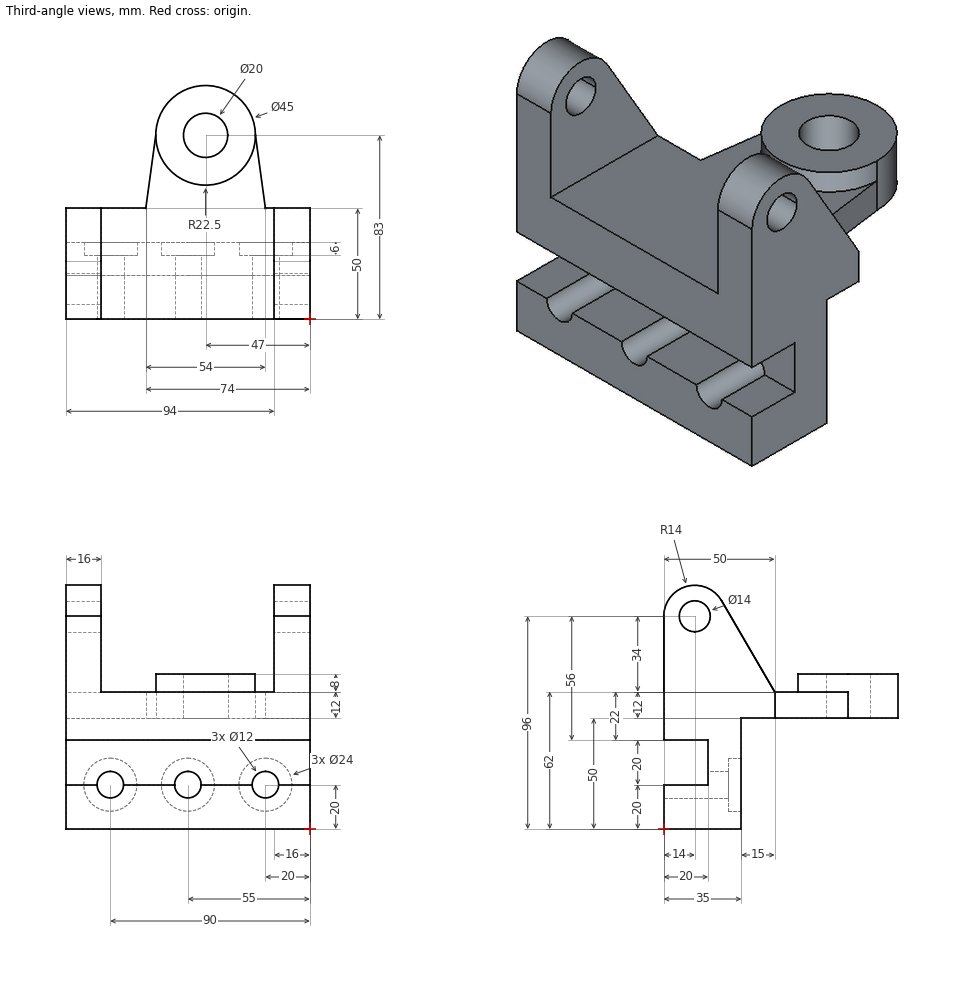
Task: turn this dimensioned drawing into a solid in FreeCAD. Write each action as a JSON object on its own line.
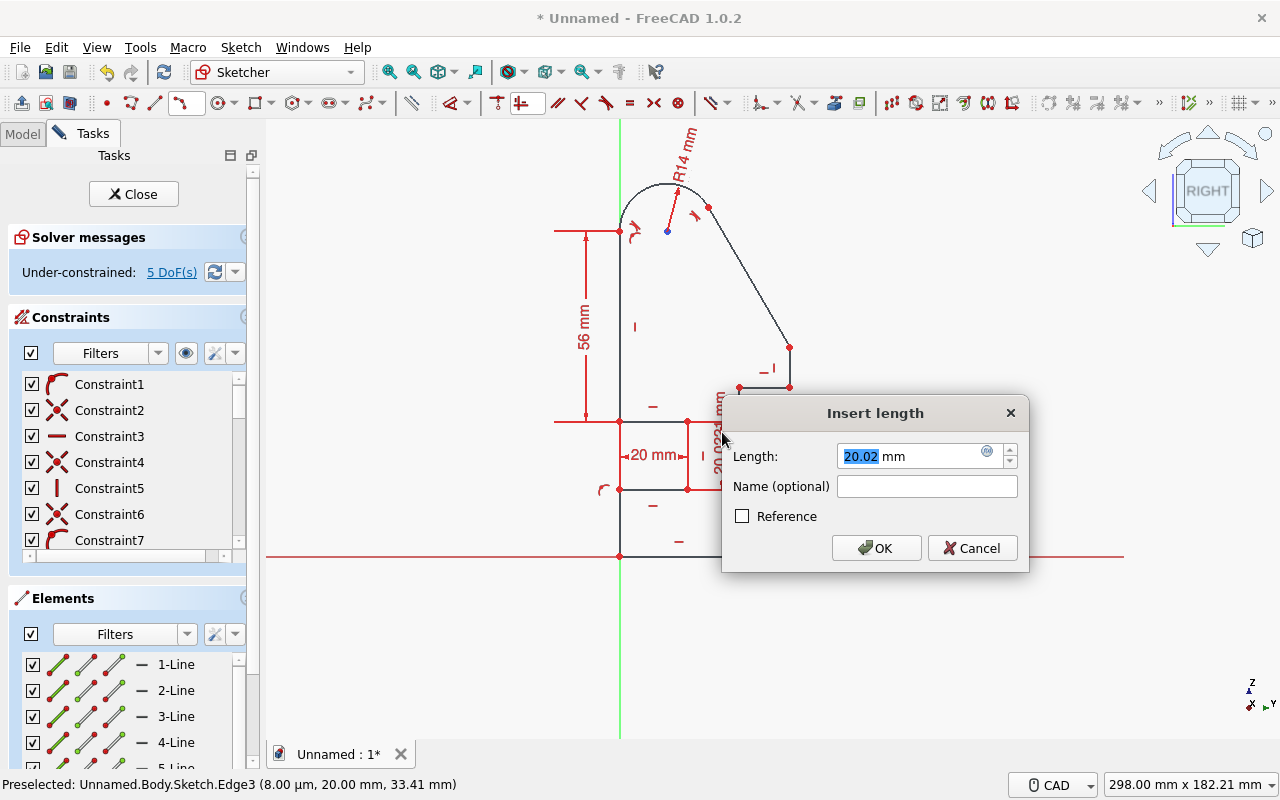
{"action": "type", "text": "20"}
{"action": "key", "text": "Return"}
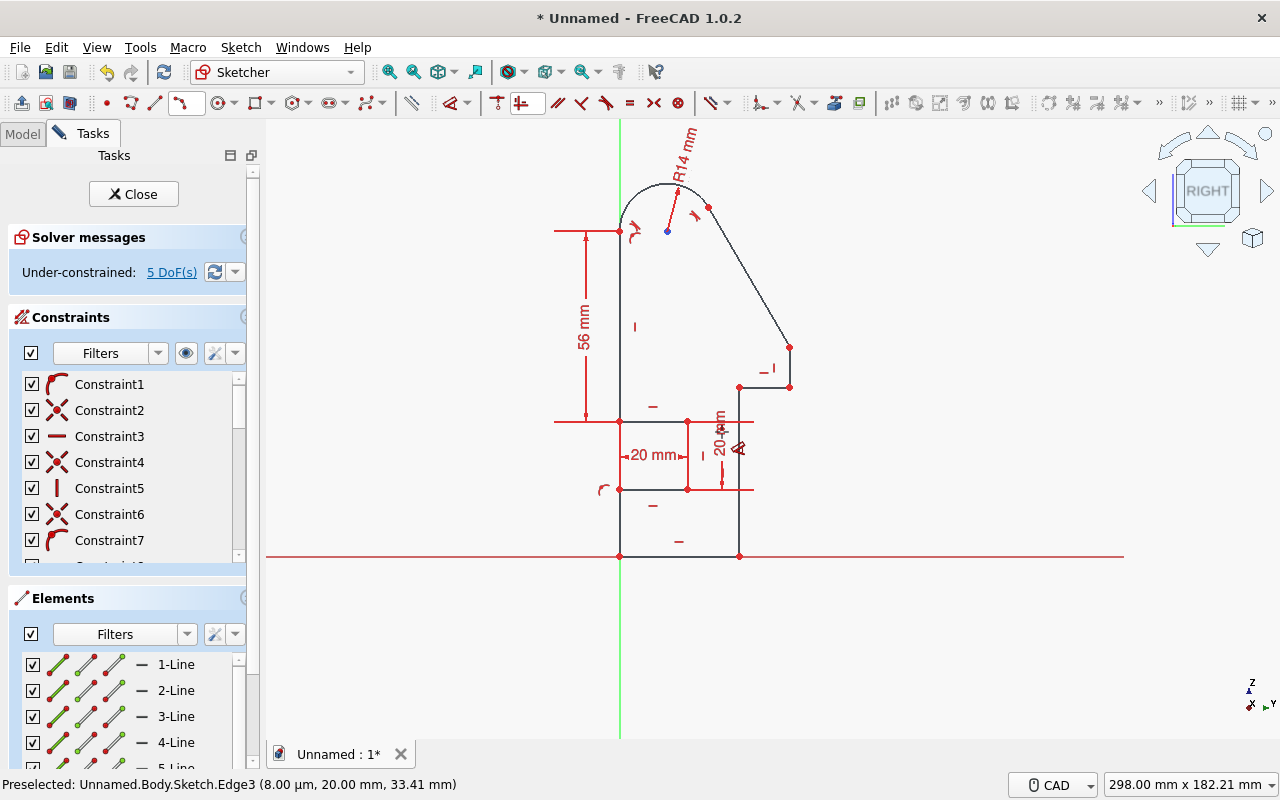
{"action": "left_click", "coordinate": [620, 510]}
{"action": "left_click", "coordinate": [586, 523]}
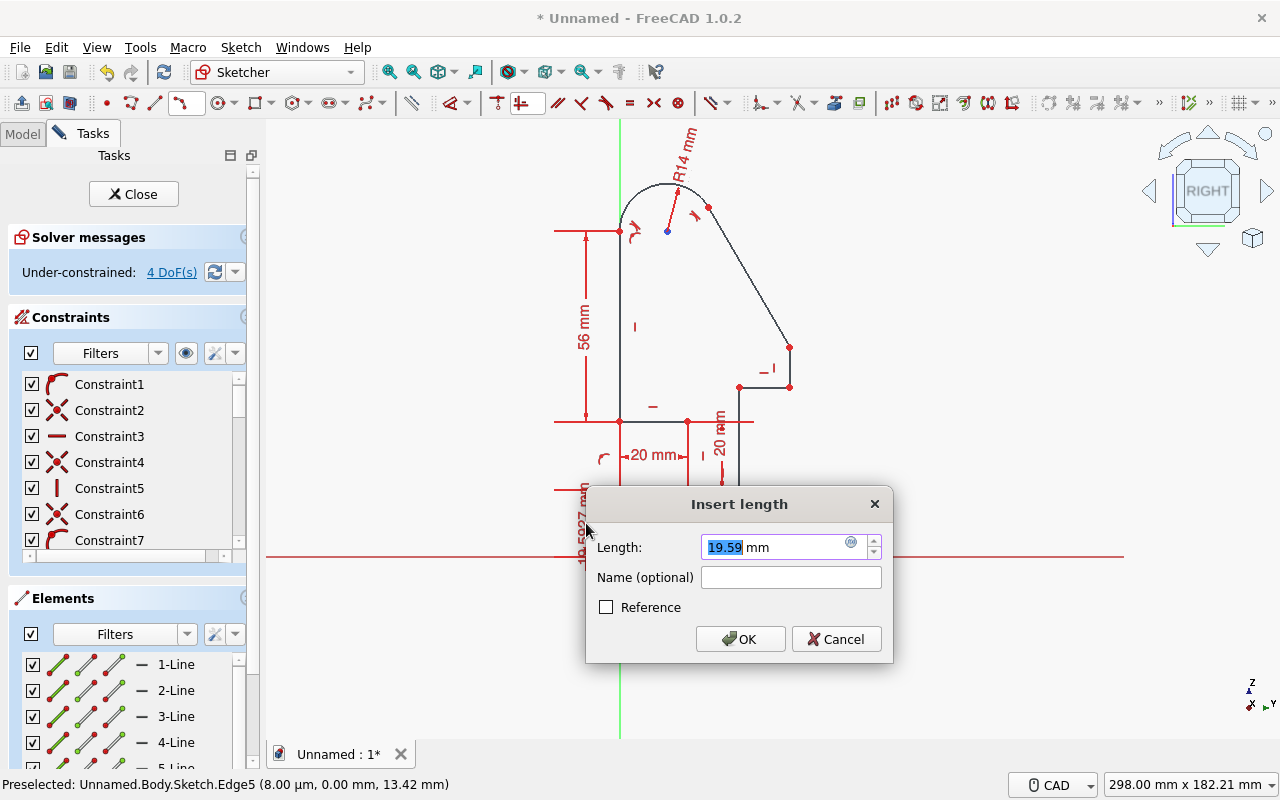
{"action": "type", "text": "20"}
{"action": "key", "text": "Return"}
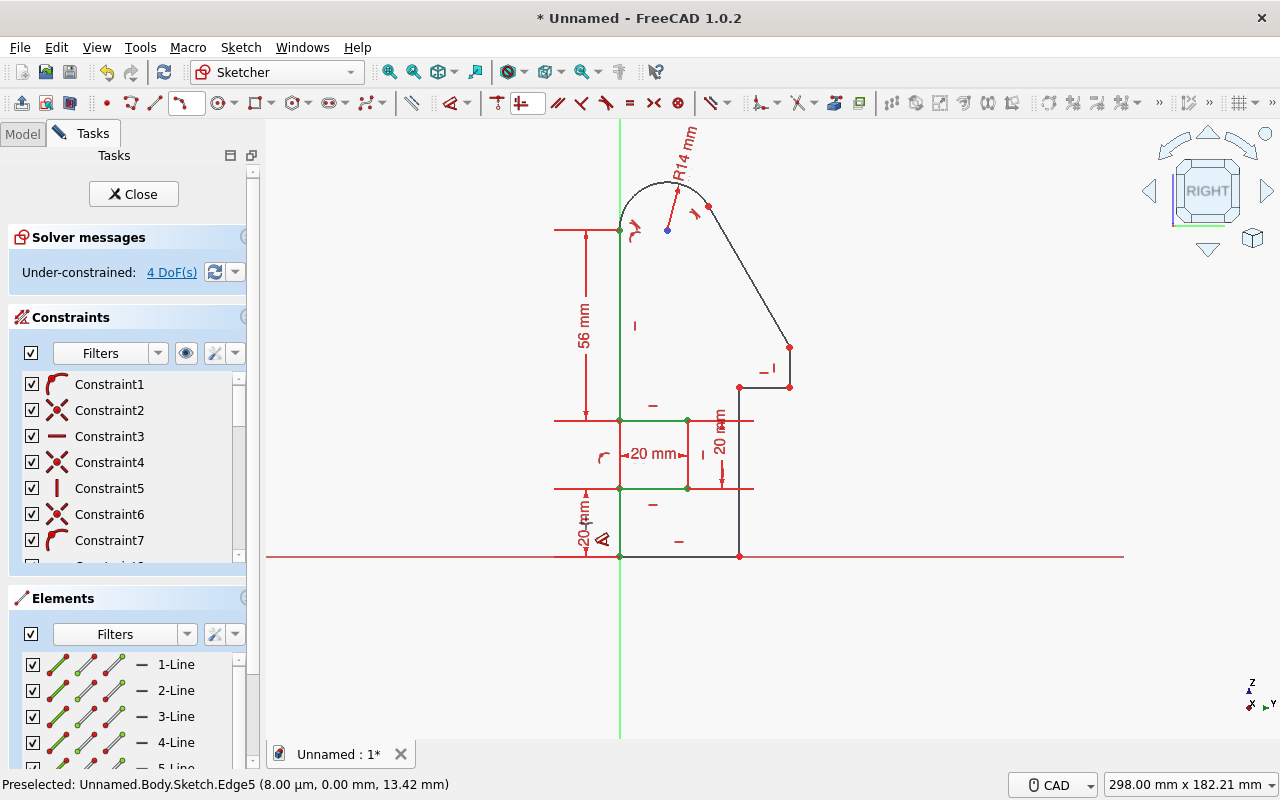
{"action": "left_click", "coordinate": [655, 557]}
{"action": "left_click", "coordinate": [679, 591]}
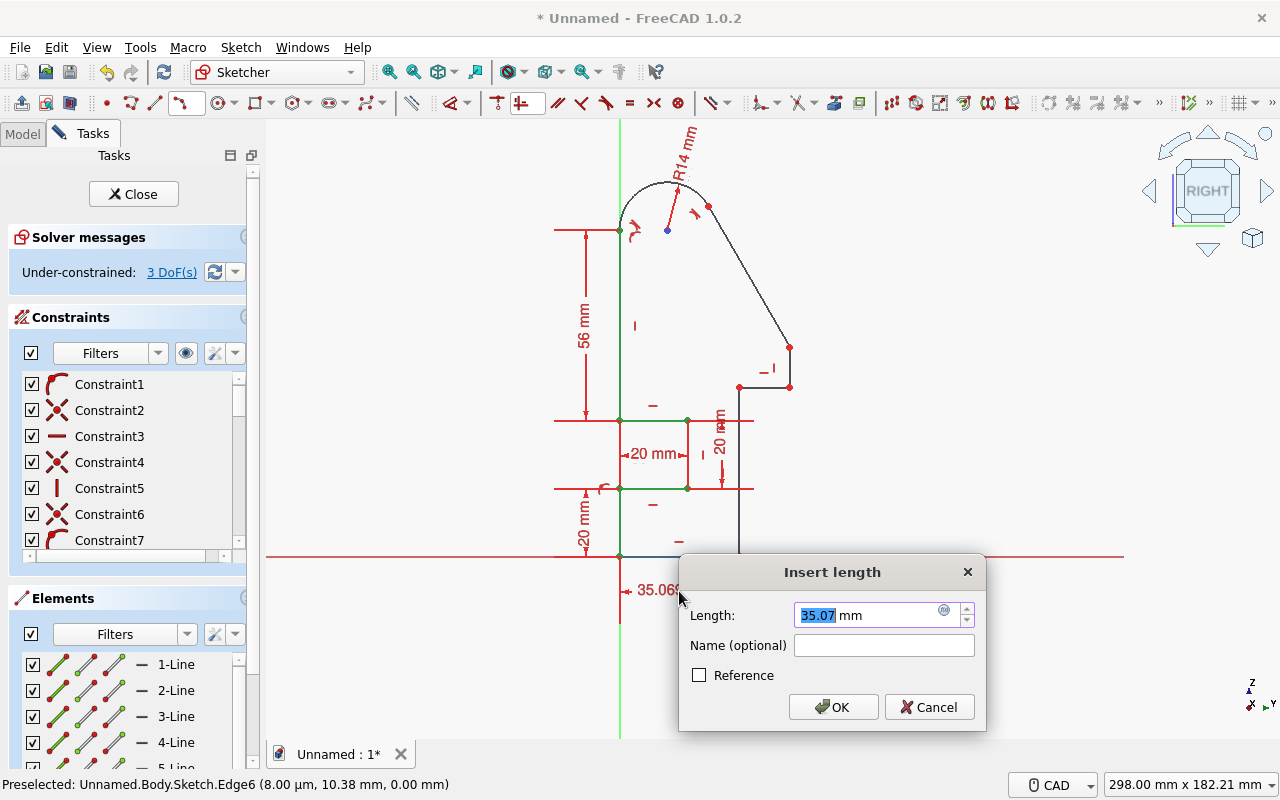
{"action": "type", "text": "35"}
{"action": "key", "text": "Return"}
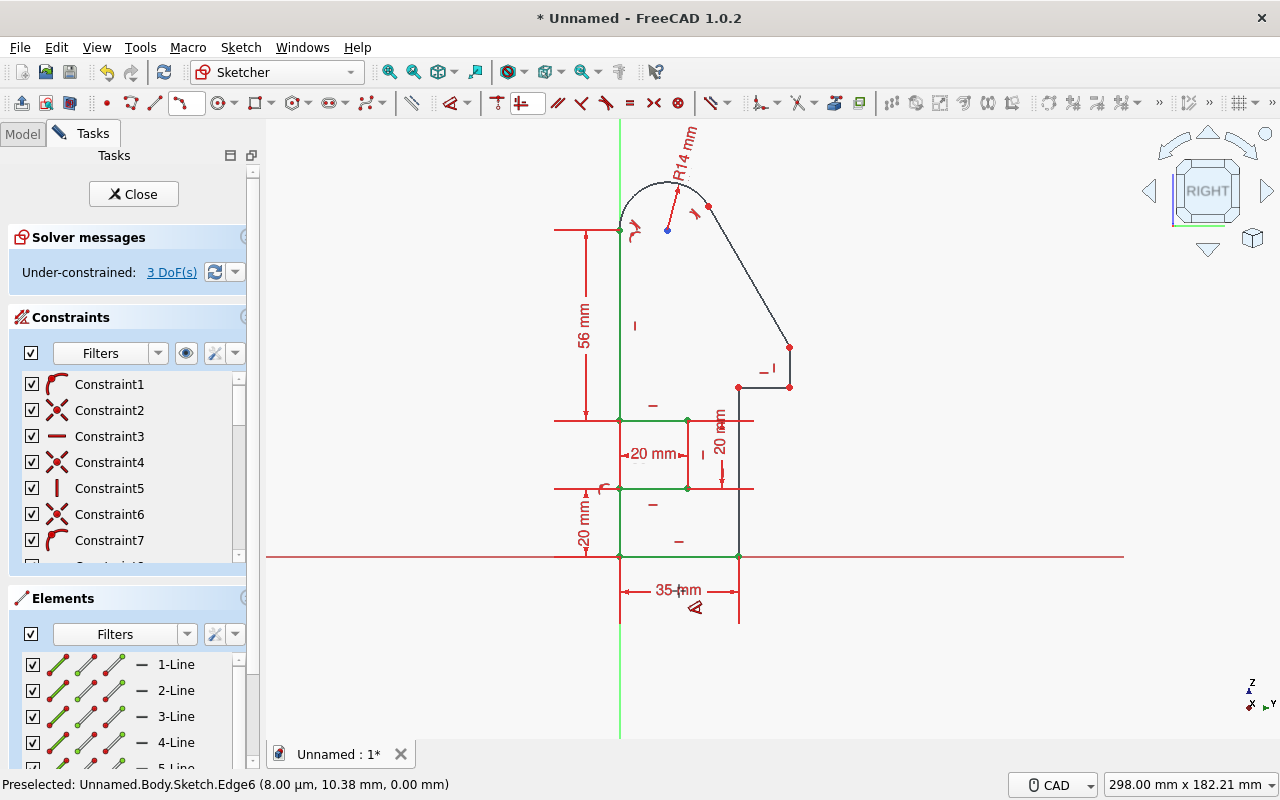
{"action": "left_click", "coordinate": [739, 506]}
{"action": "left_click", "coordinate": [773, 472]}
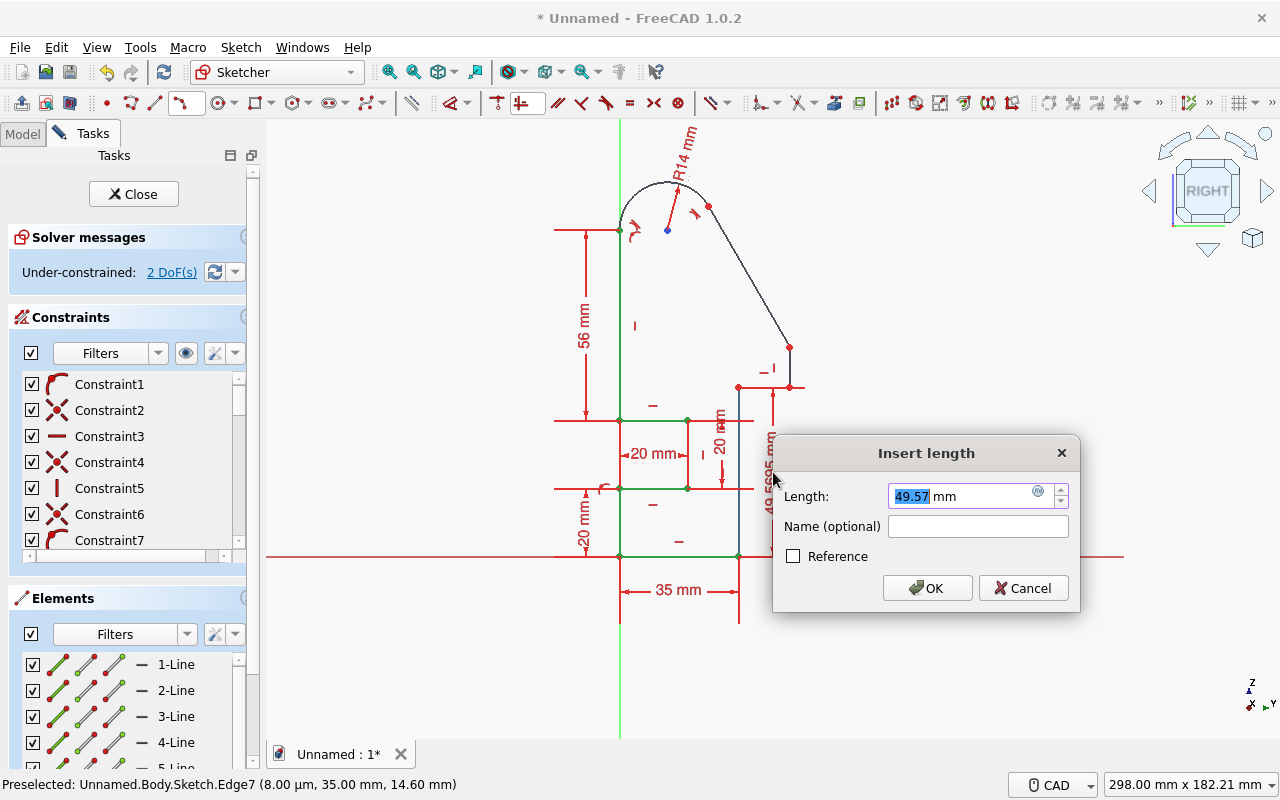
{"action": "type", "text": "50"}
{"action": "key", "text": "Return"}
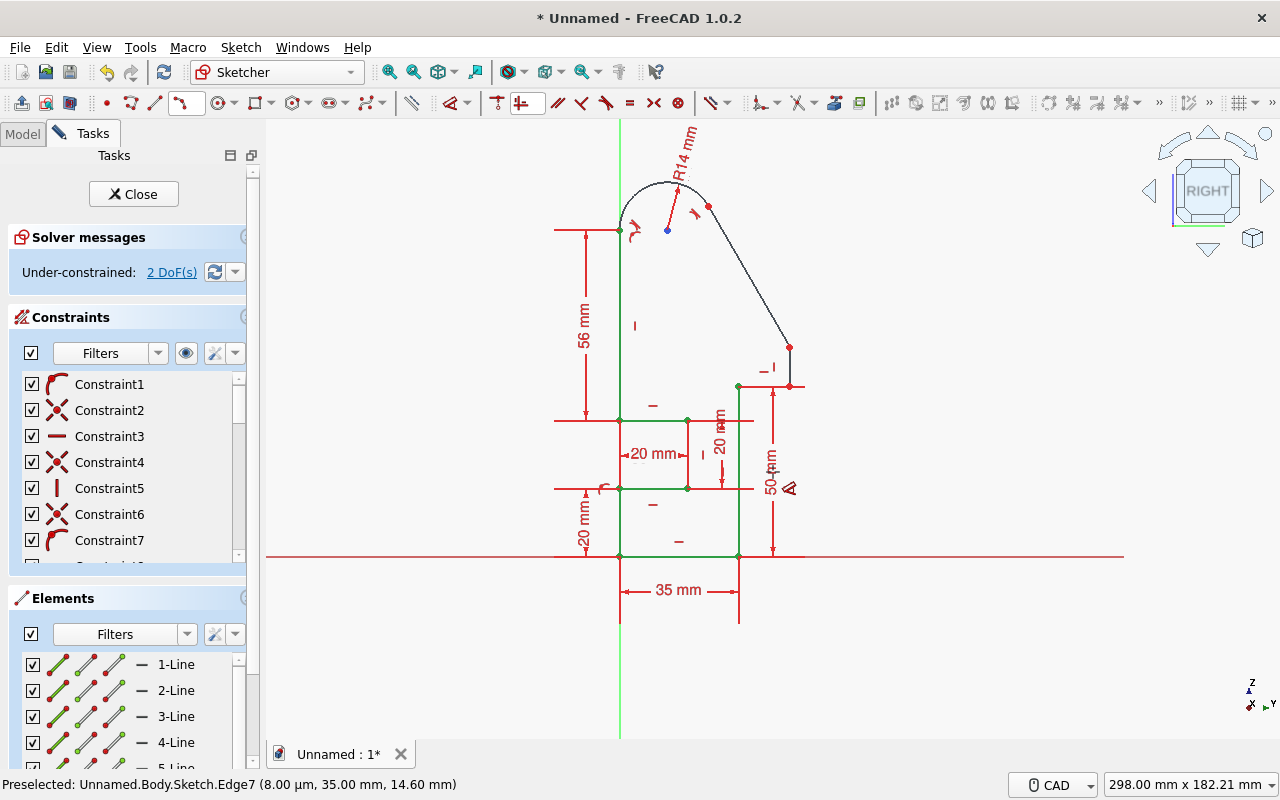
{"action": "left_click", "coordinate": [754, 387]}
{"action": "left_click", "coordinate": [764, 353]}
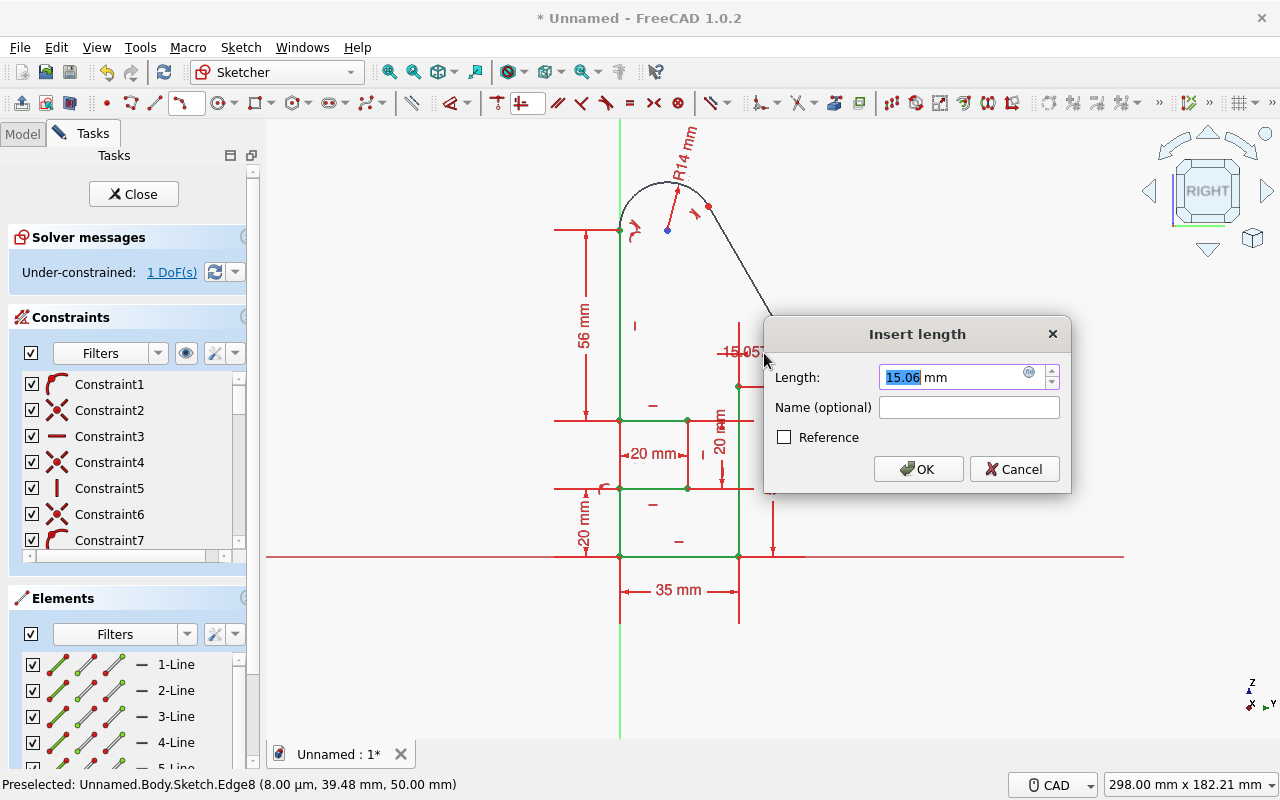
{"action": "type", "text": "15"}
{"action": "key", "text": "Return"}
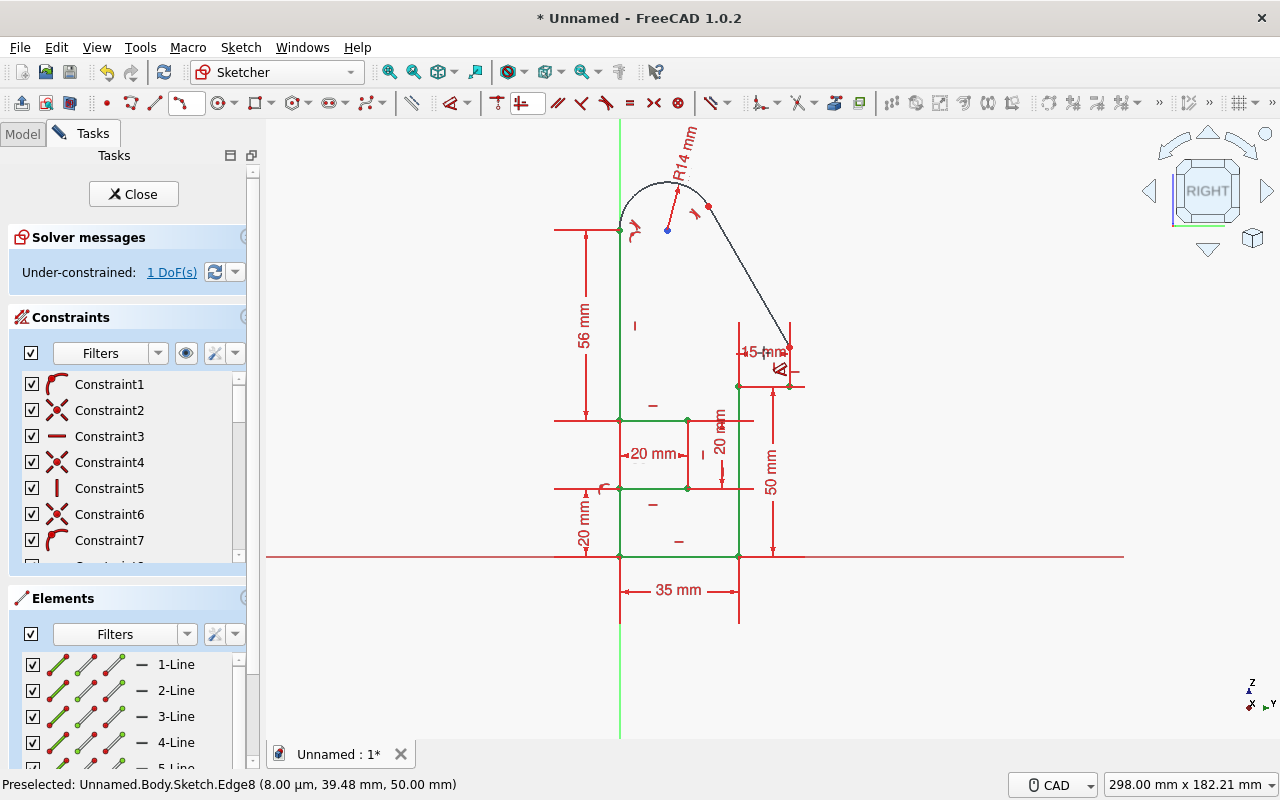
{"action": "left_click", "coordinate": [790, 375]}
{"action": "left_click", "coordinate": [824, 376]}